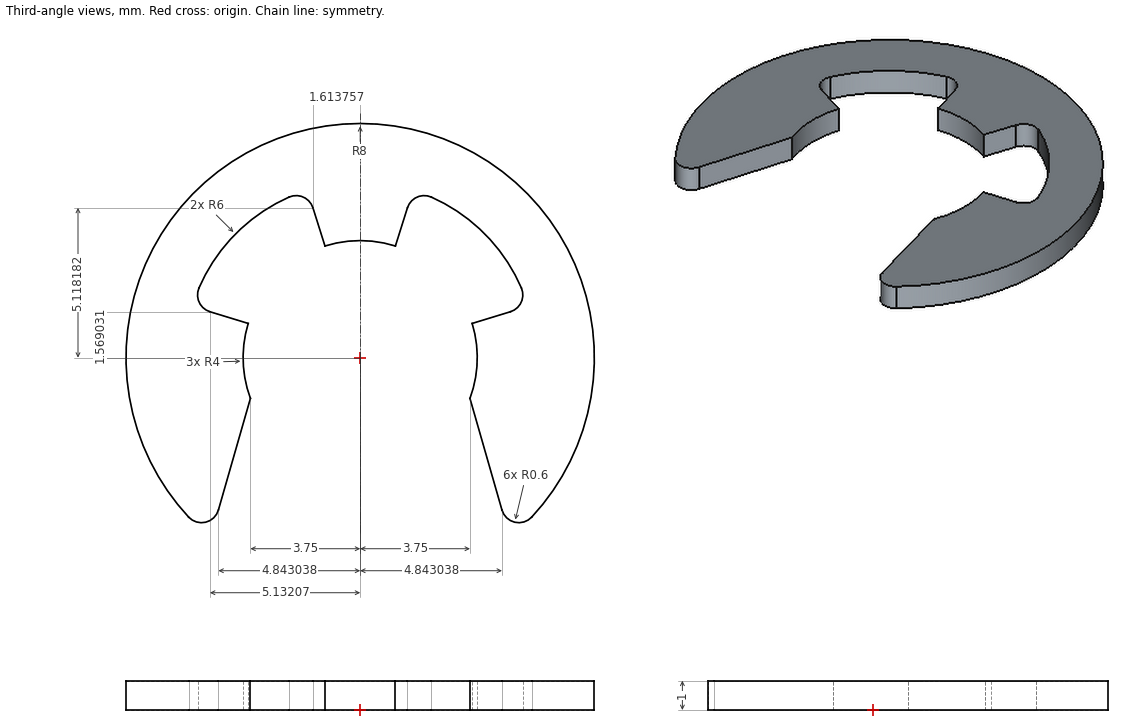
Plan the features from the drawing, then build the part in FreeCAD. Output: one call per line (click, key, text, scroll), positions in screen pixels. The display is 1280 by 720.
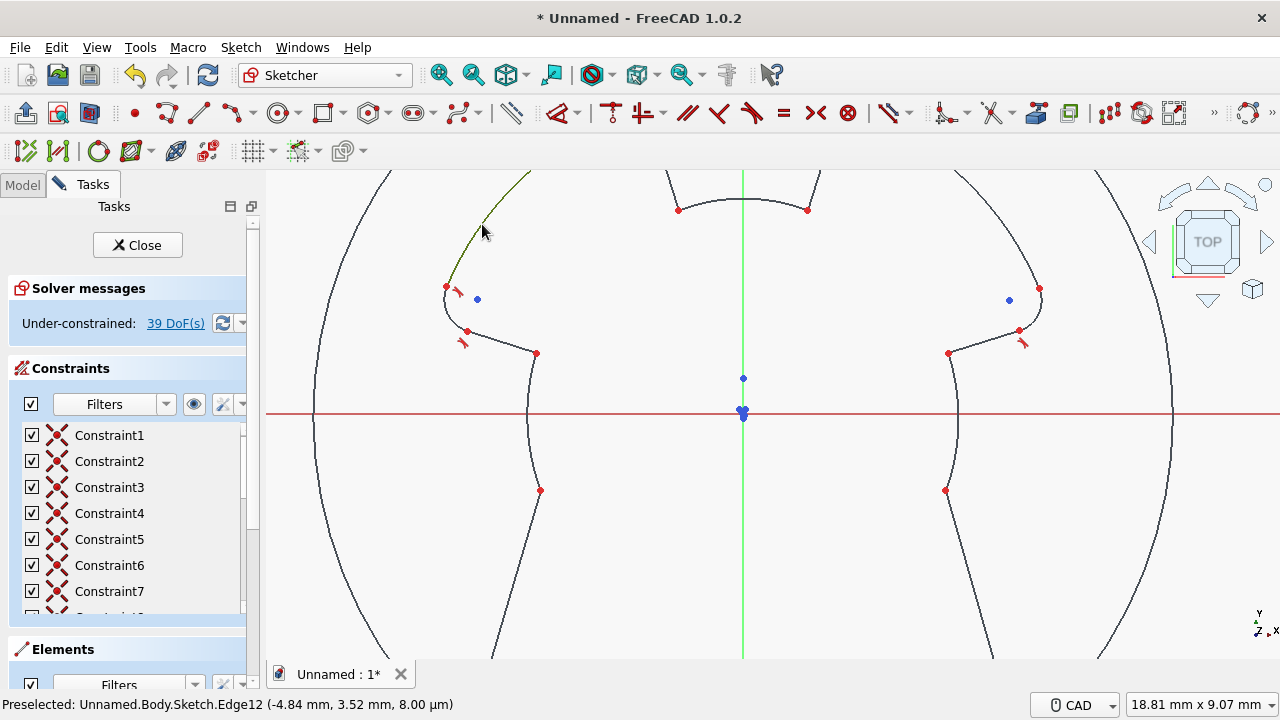
scroll(673, 468, down, 4)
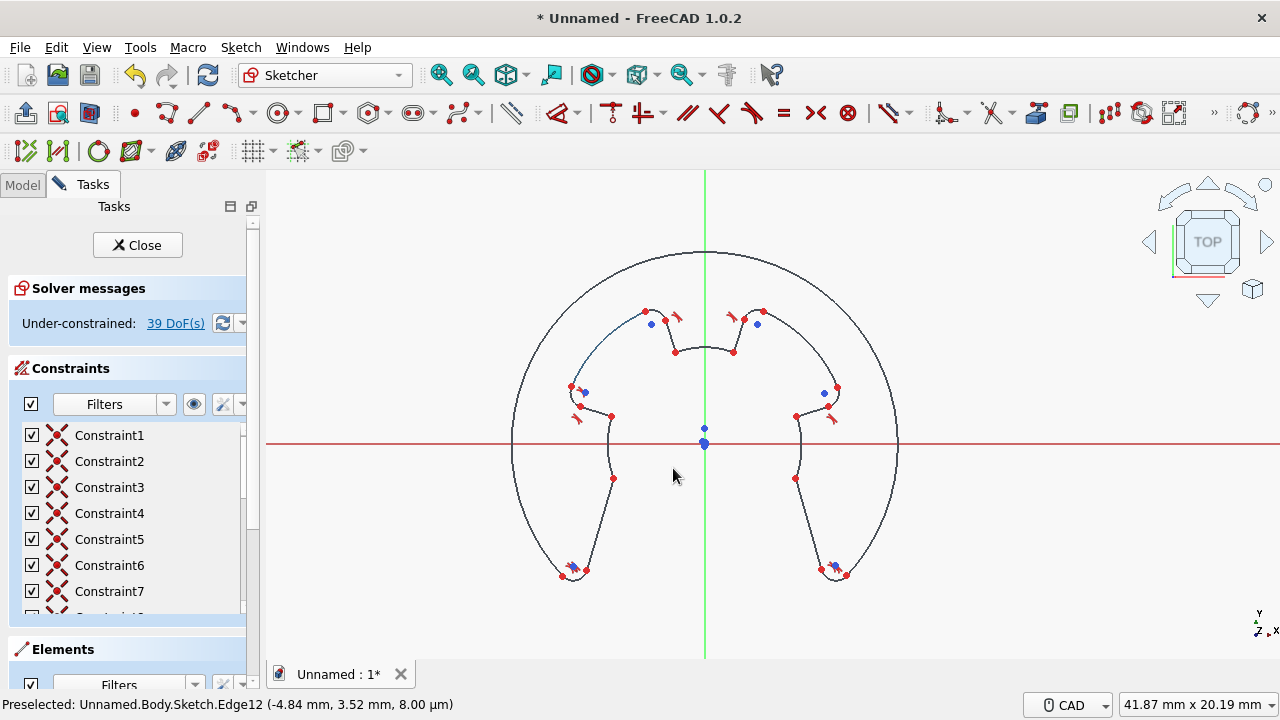
scroll(662, 314, up, 4)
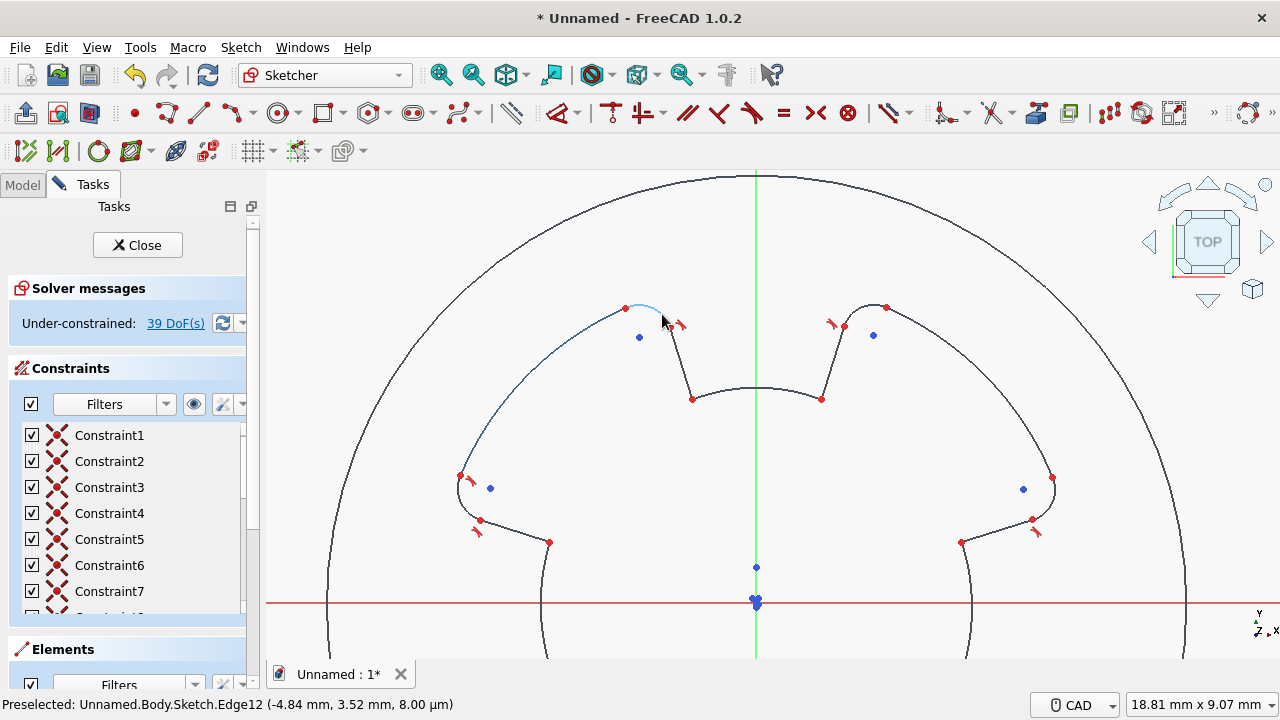
click(661, 314)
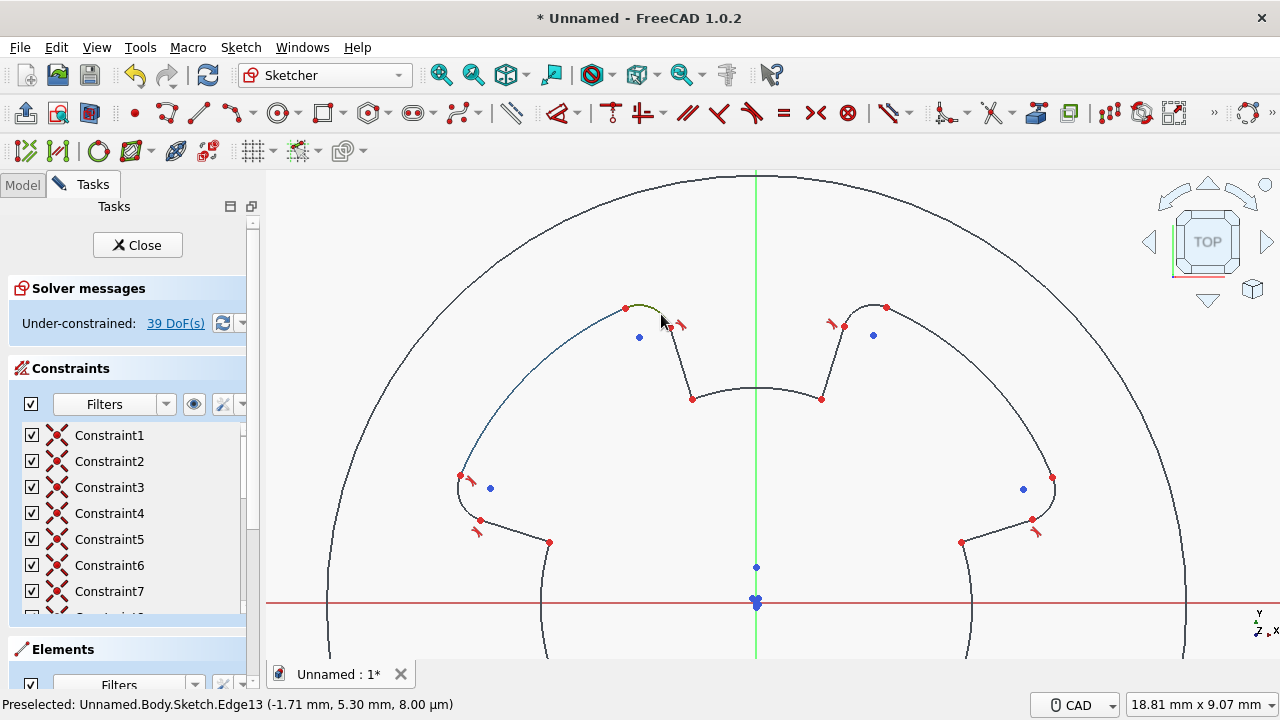
key(t)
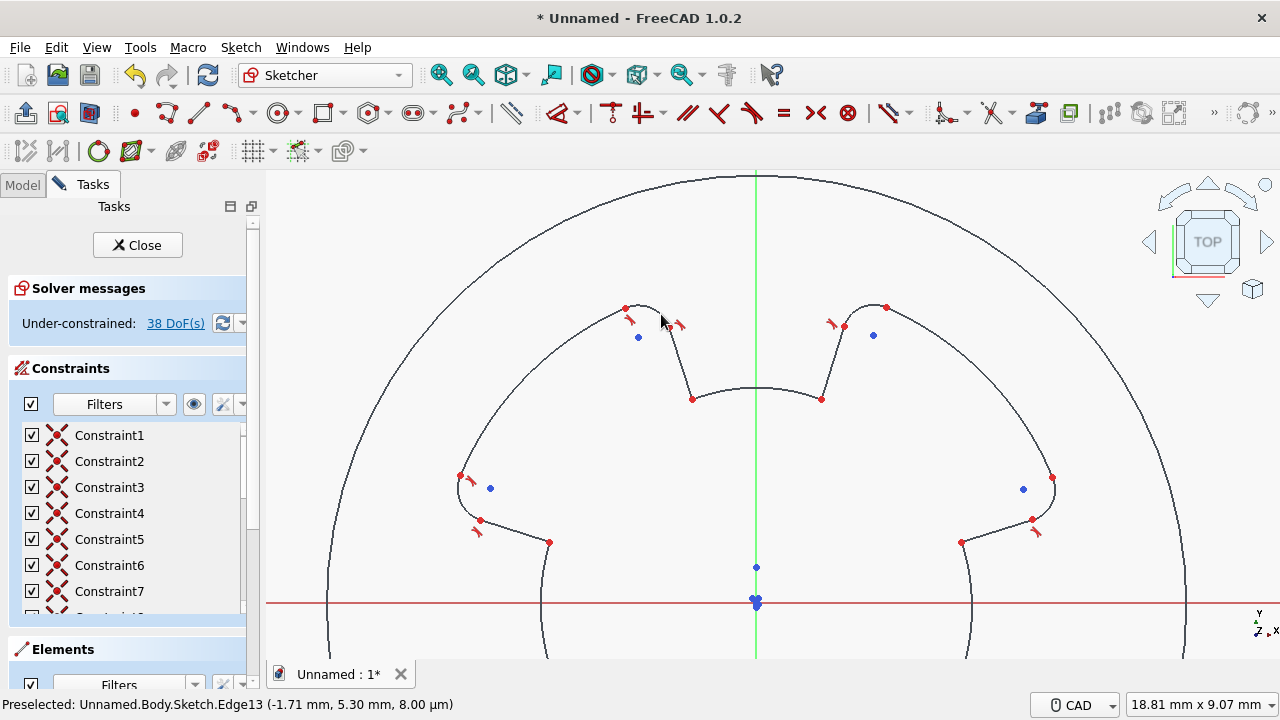
click(872, 305)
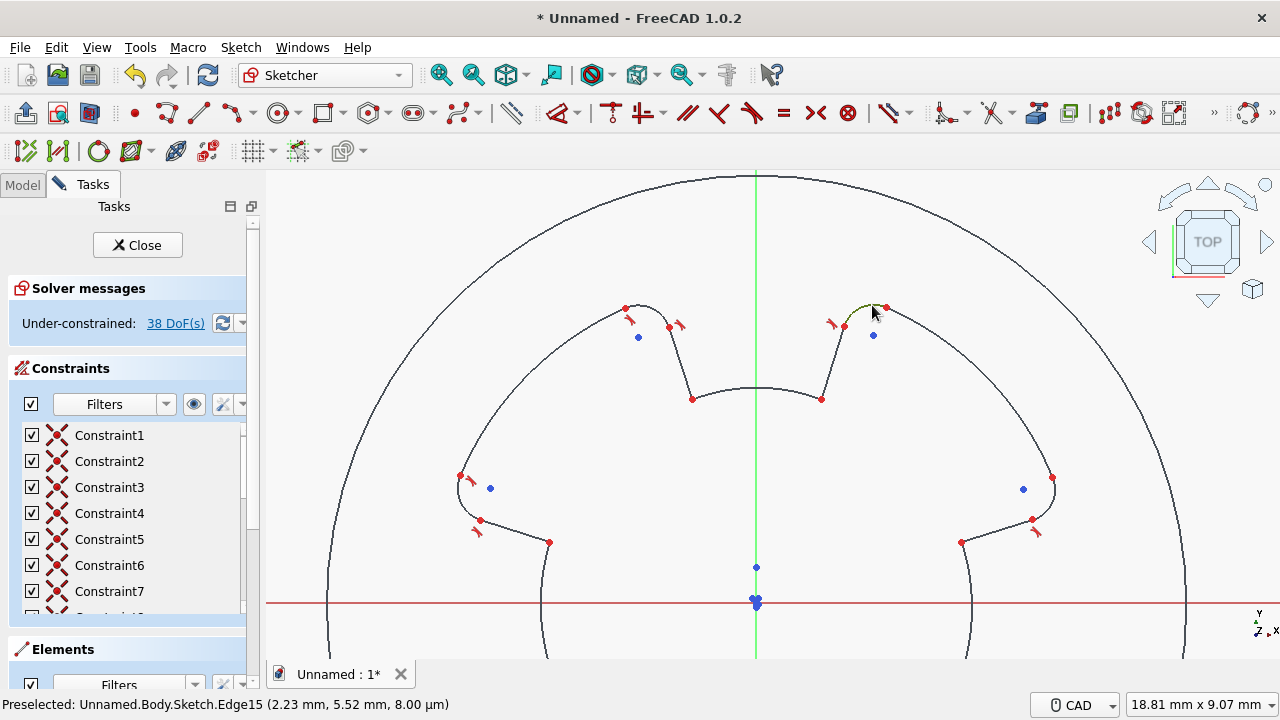
click(1017, 414)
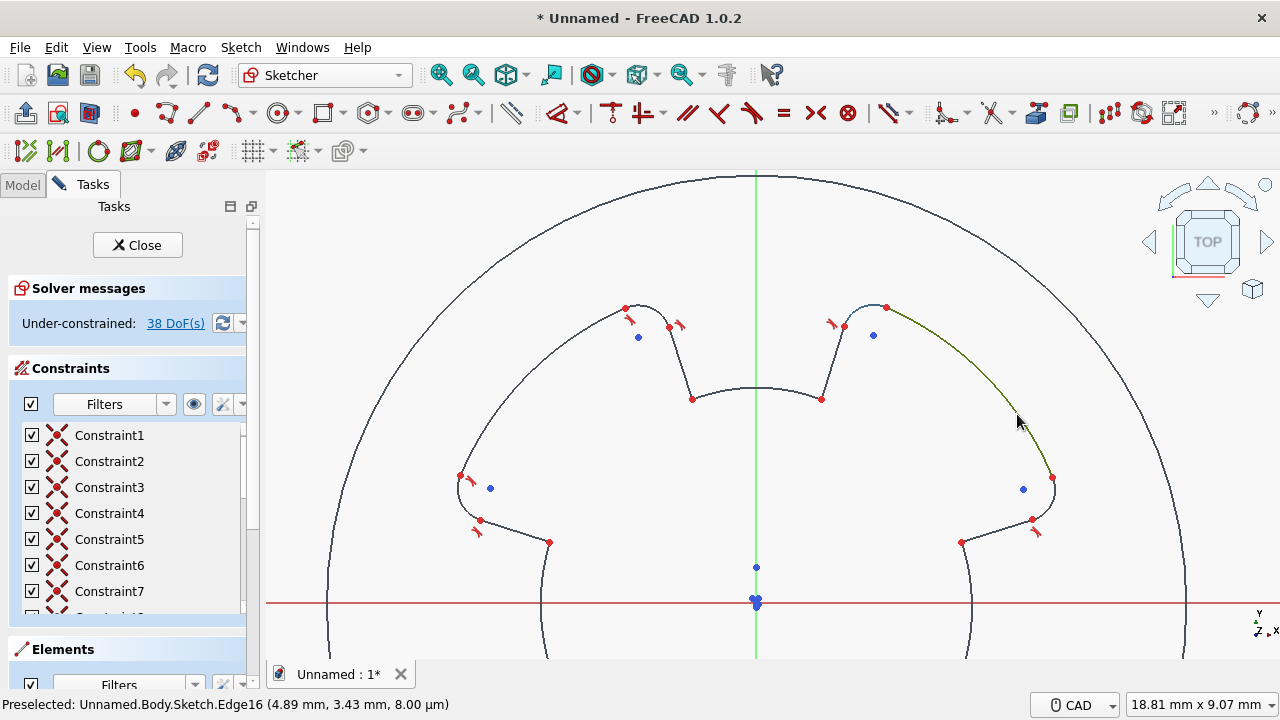
key(t)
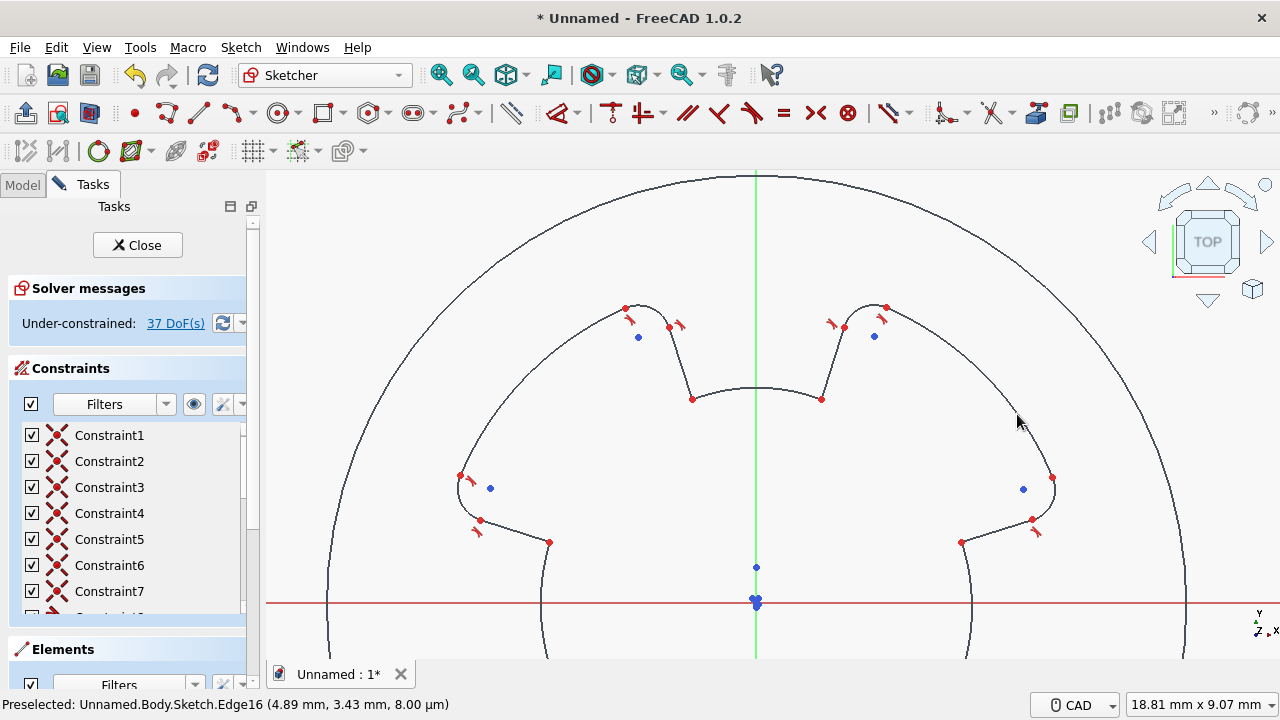
click(1017, 414)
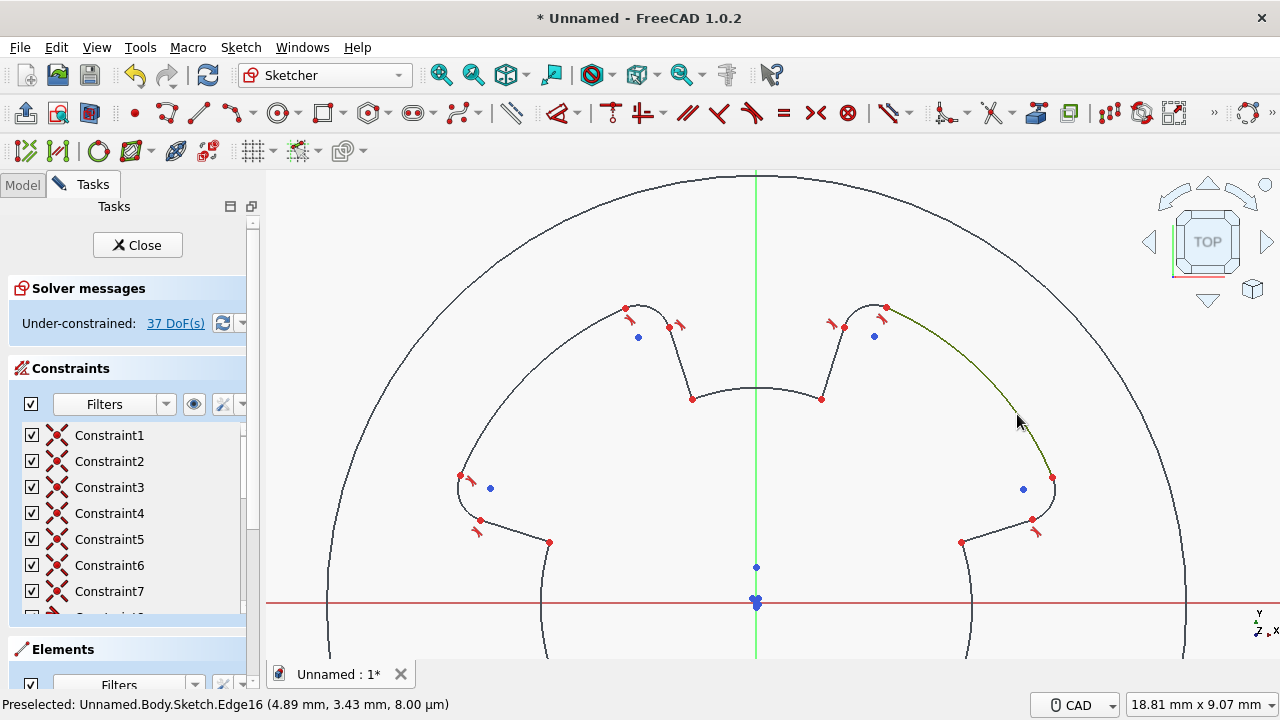
click(1046, 512)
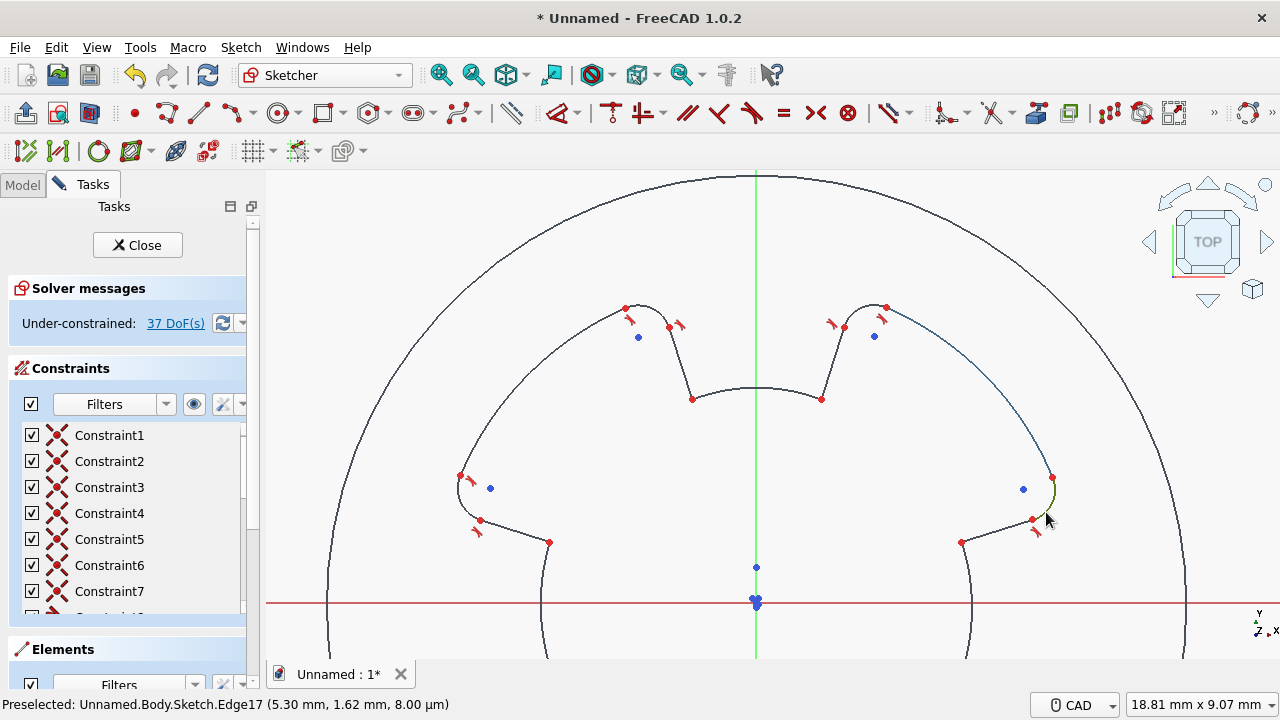
click(752, 114)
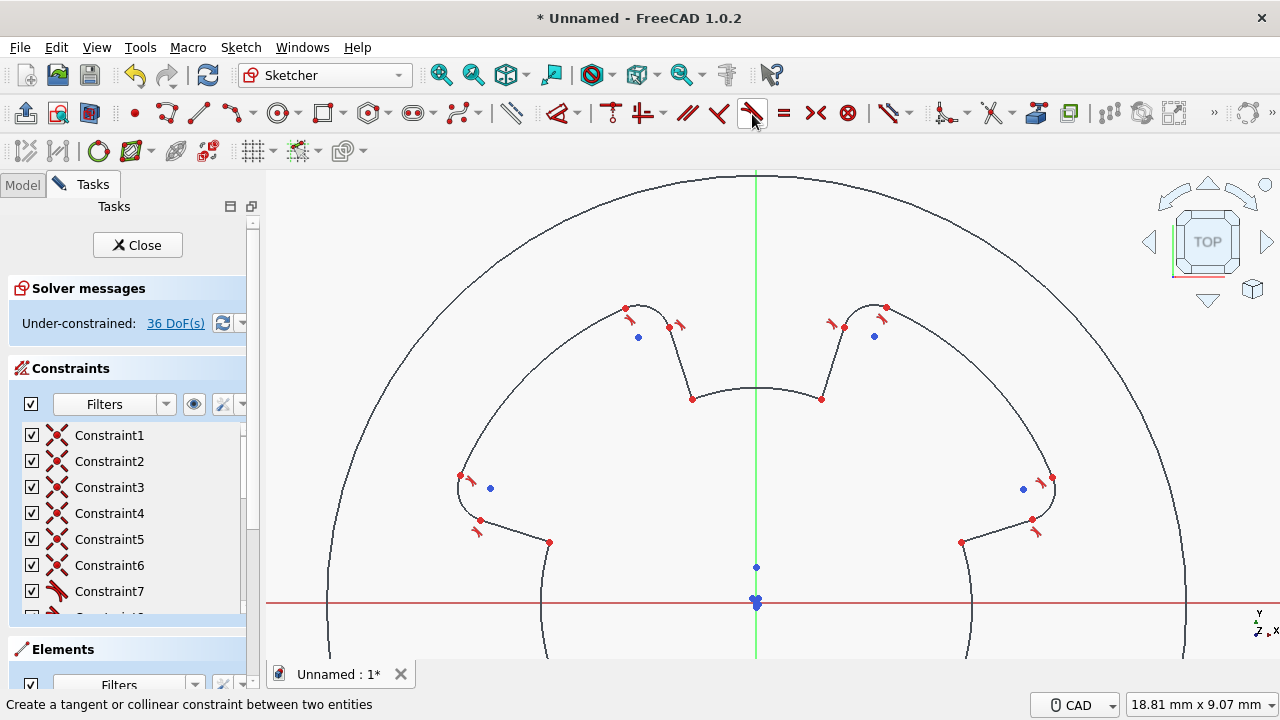
click(1100, 347)